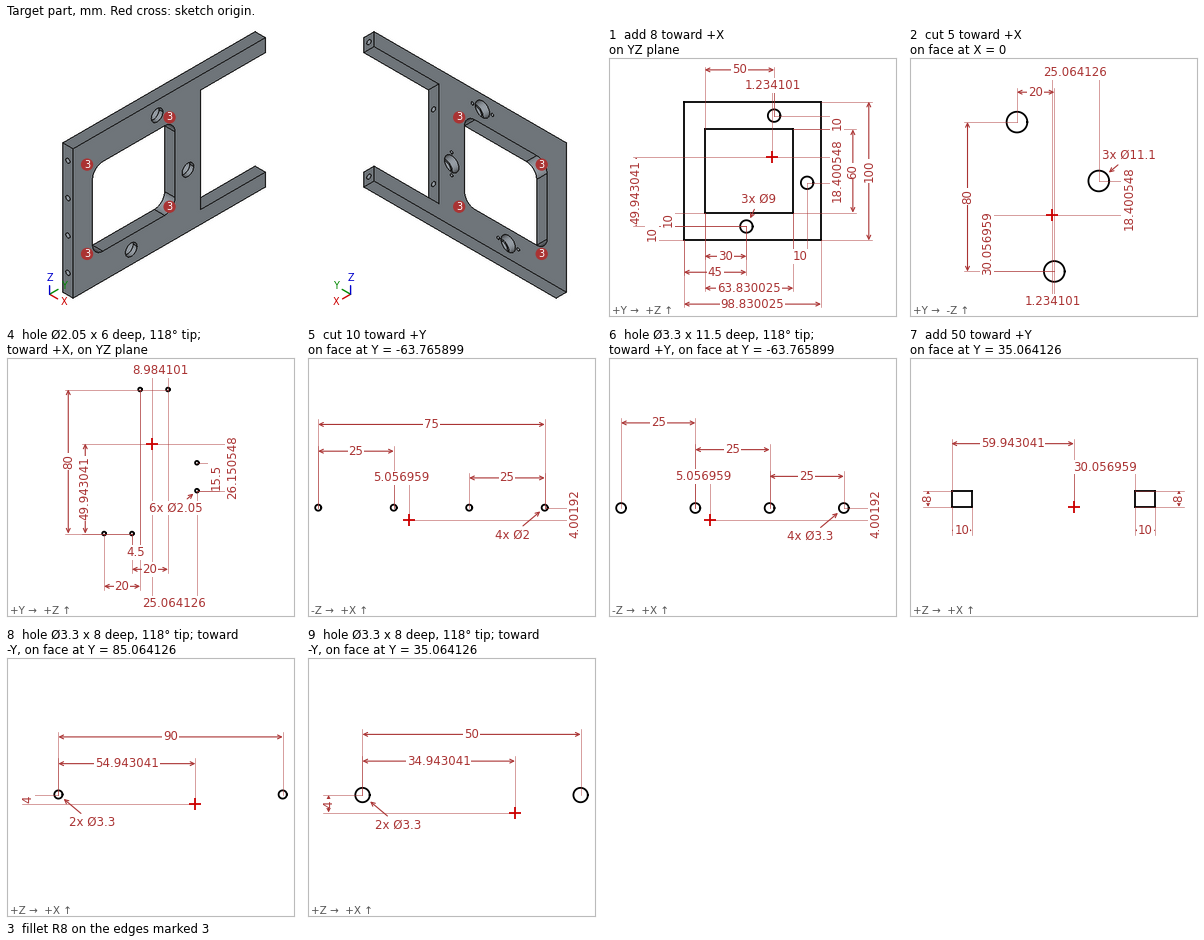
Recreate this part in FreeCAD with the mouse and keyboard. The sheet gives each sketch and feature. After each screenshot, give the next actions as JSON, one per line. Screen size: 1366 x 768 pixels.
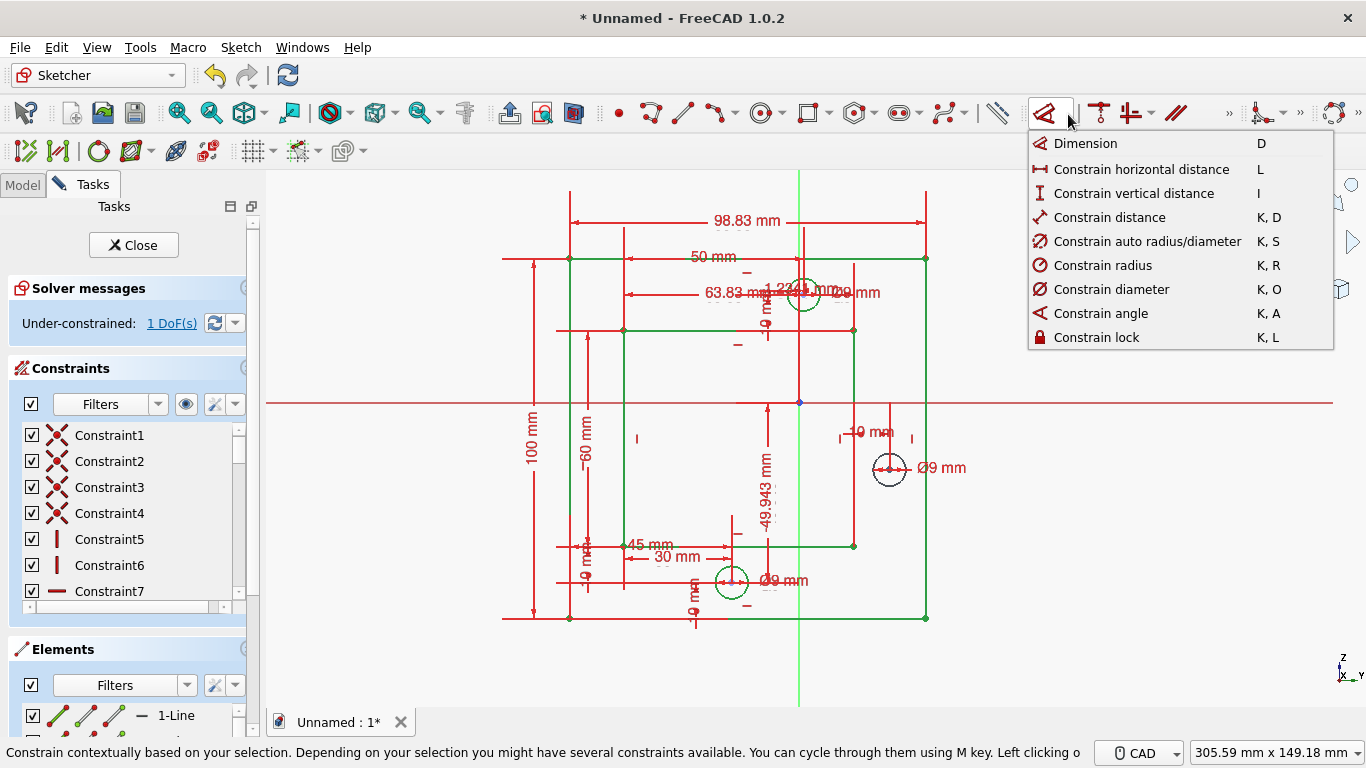
{"action": "left_click", "coordinate": [1181, 193]}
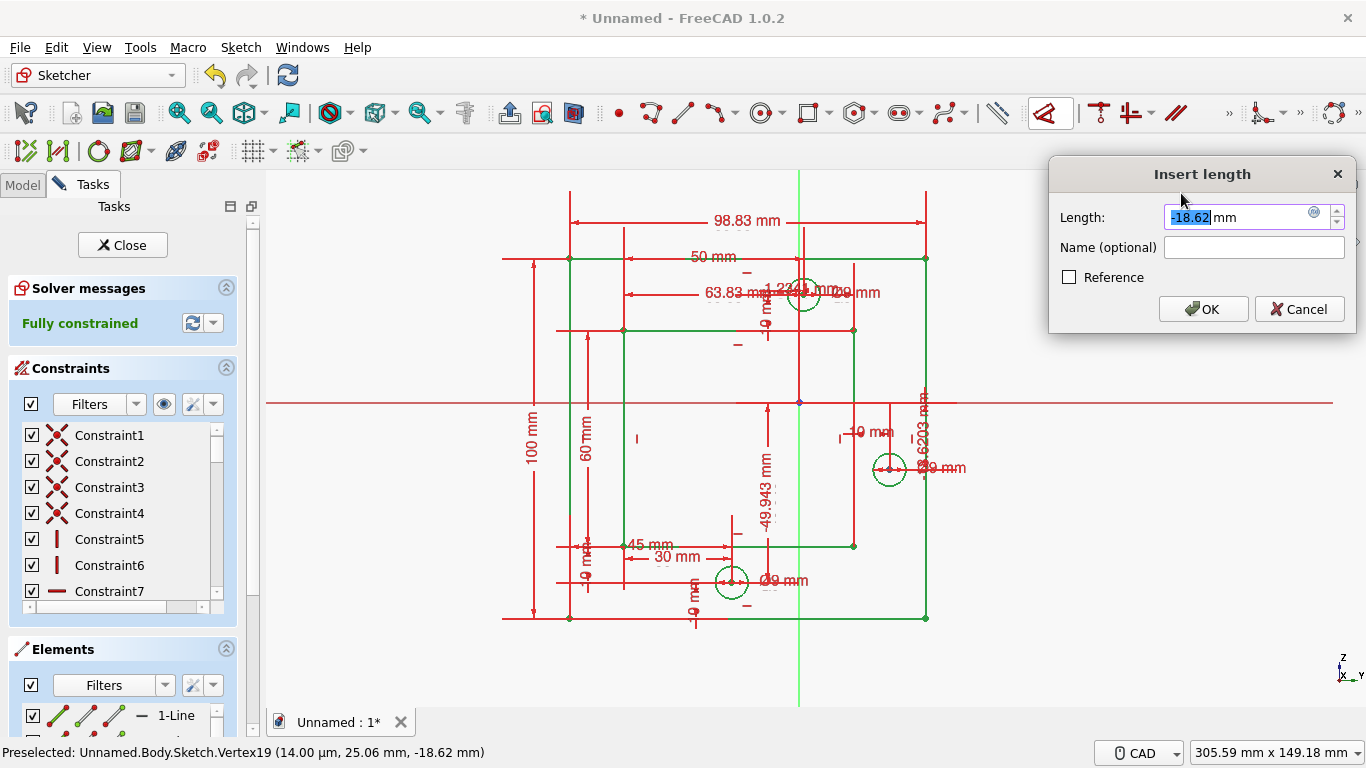
{"action": "type", "text": "-18.400548"}
{"action": "key", "text": "Return"}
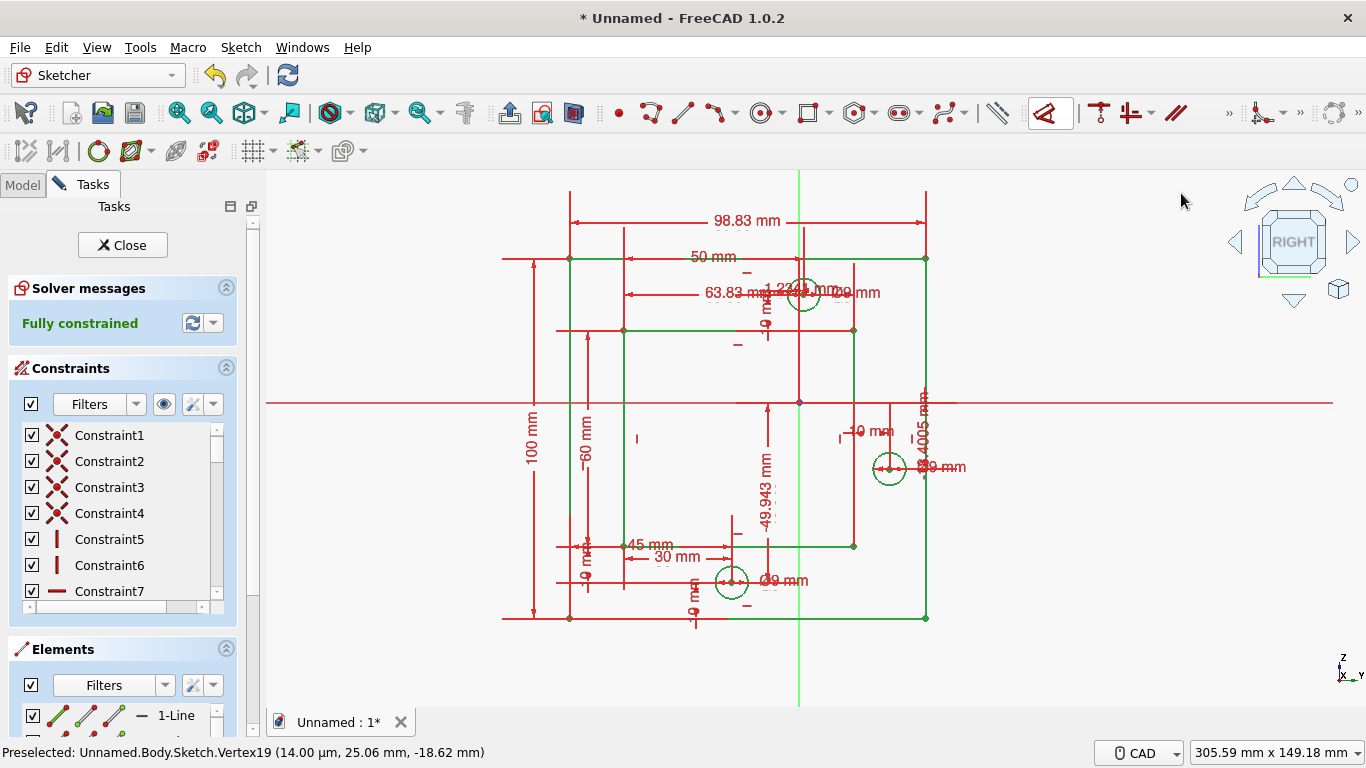
{"action": "left_click", "coordinate": [123, 245]}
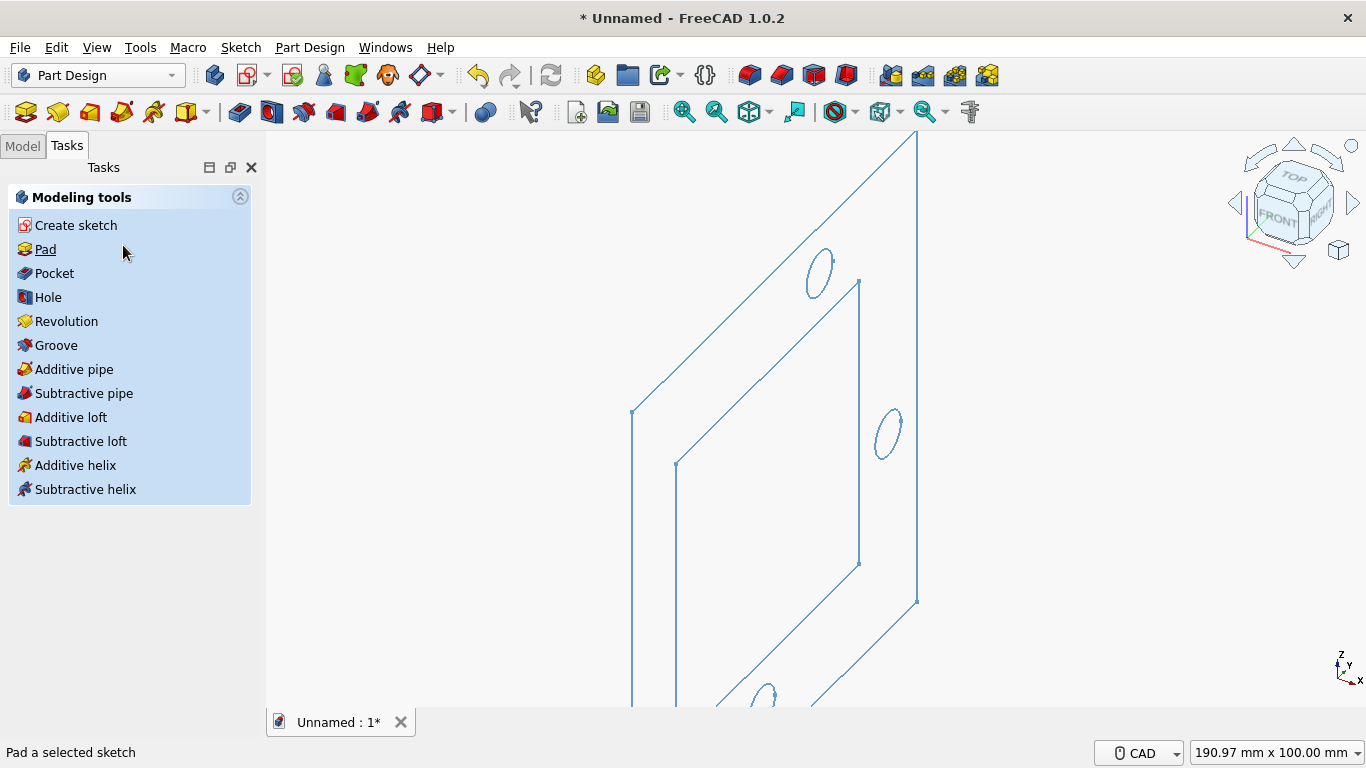
{"action": "left_click", "coordinate": [26, 112]}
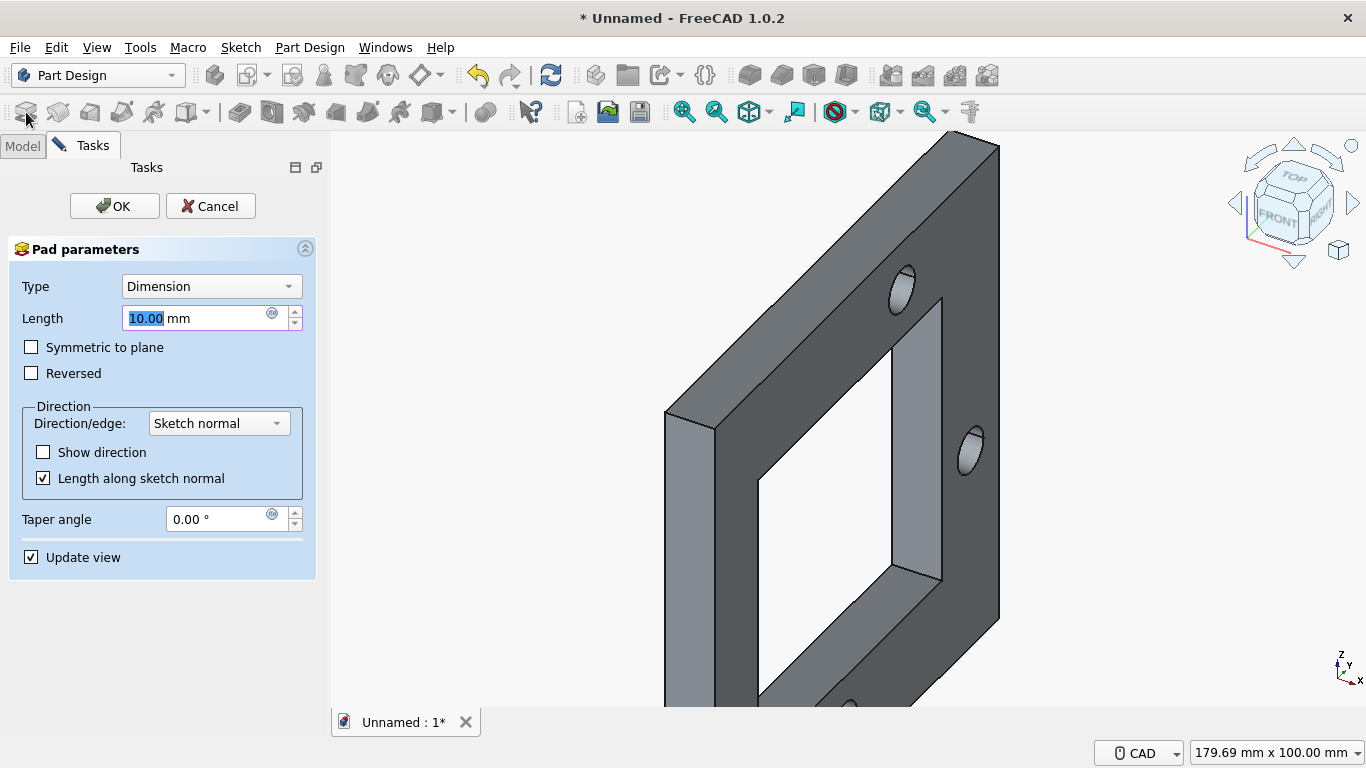
{"action": "type", "text": "8"}
{"action": "key", "text": "Tab"}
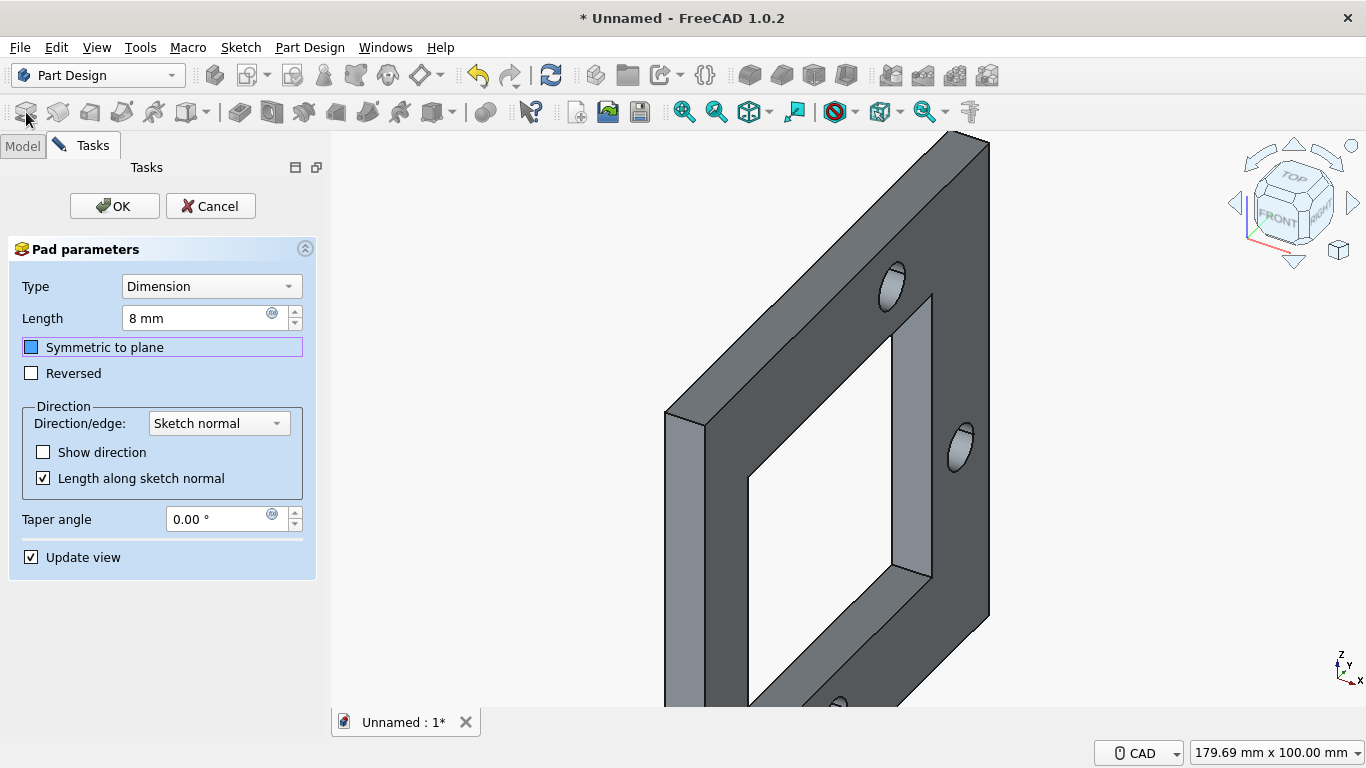
{"action": "left_click", "coordinate": [115, 206]}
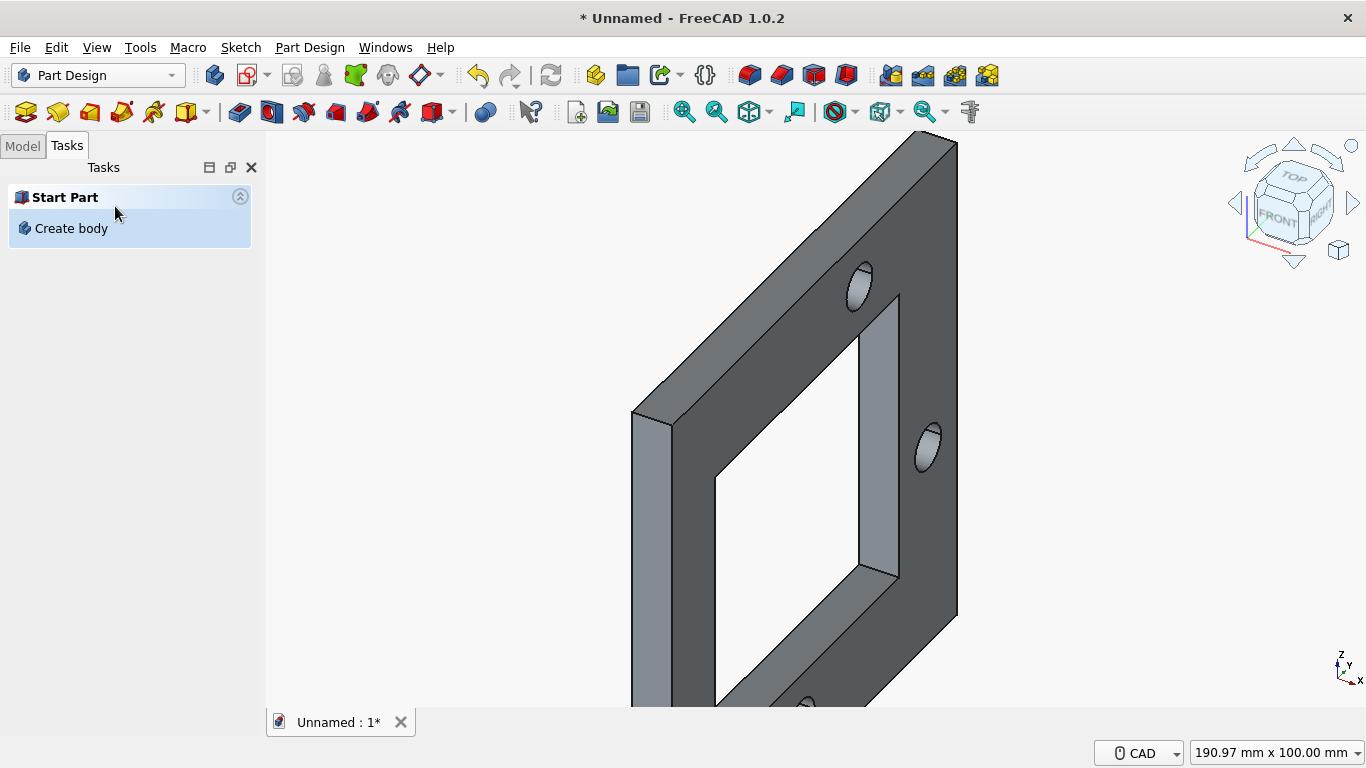
{"action": "key", "text": "v f"}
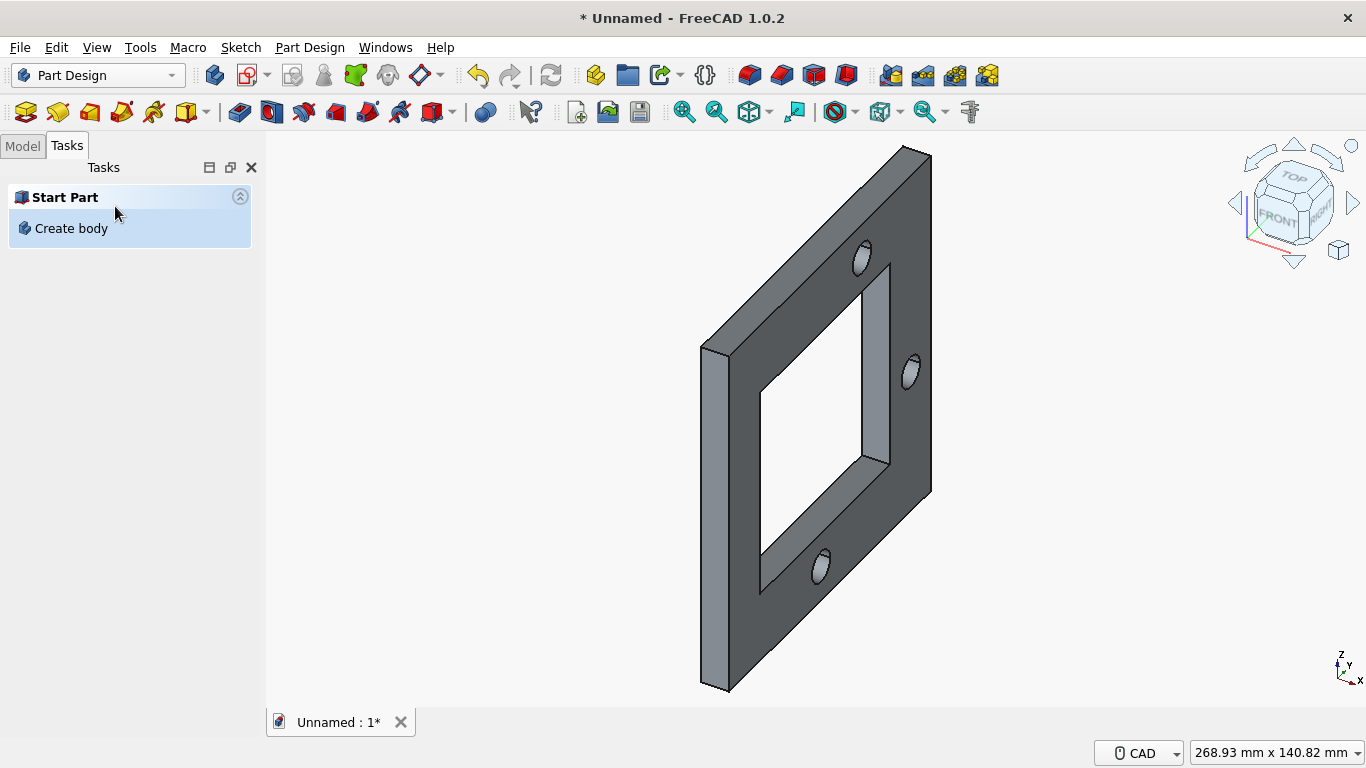
{"action": "key", "text": "6"}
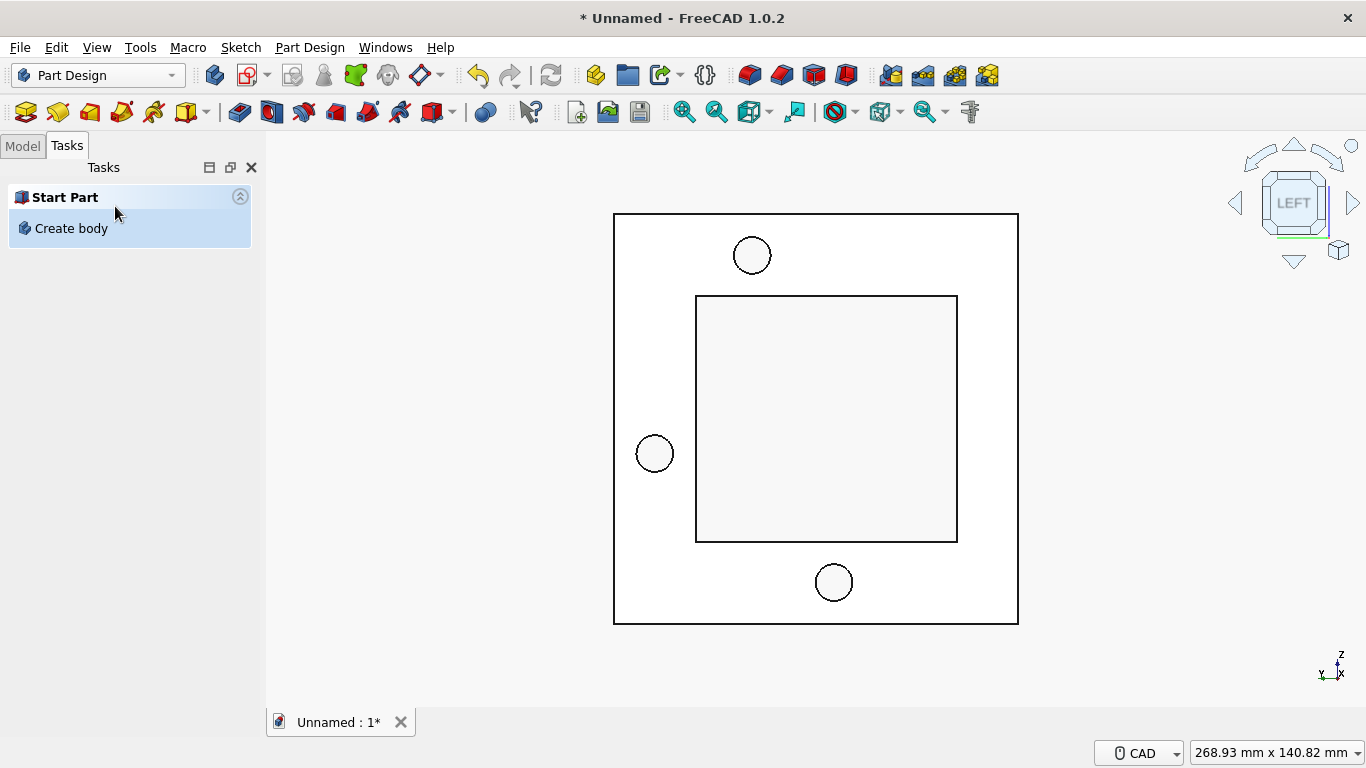
{"action": "left_click", "coordinate": [701, 593]}